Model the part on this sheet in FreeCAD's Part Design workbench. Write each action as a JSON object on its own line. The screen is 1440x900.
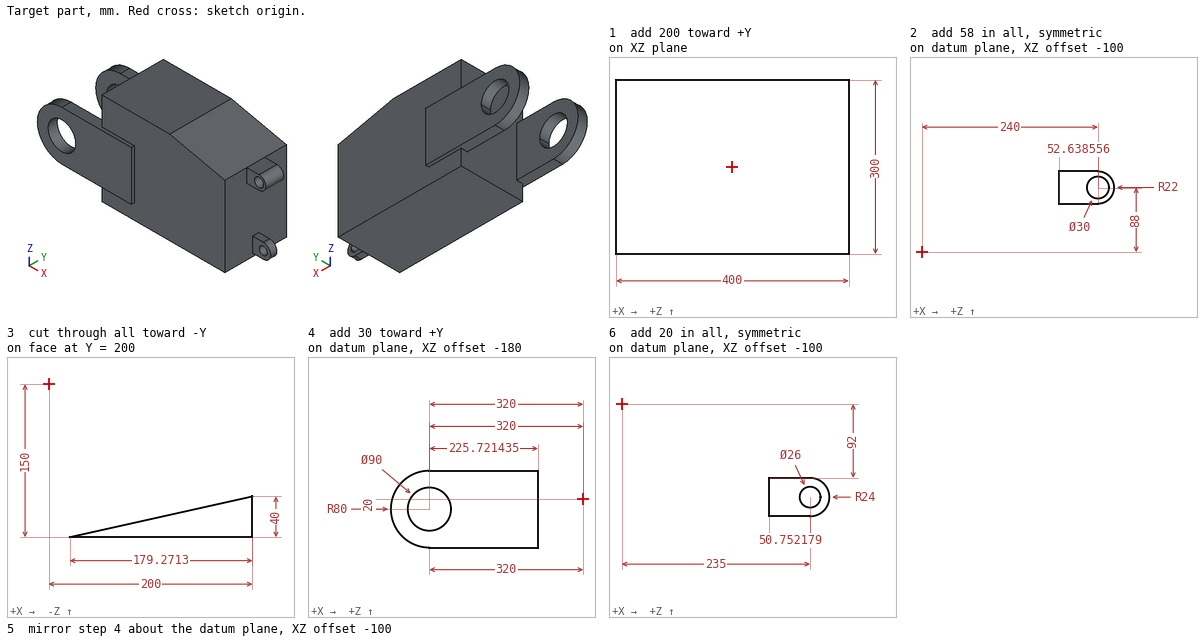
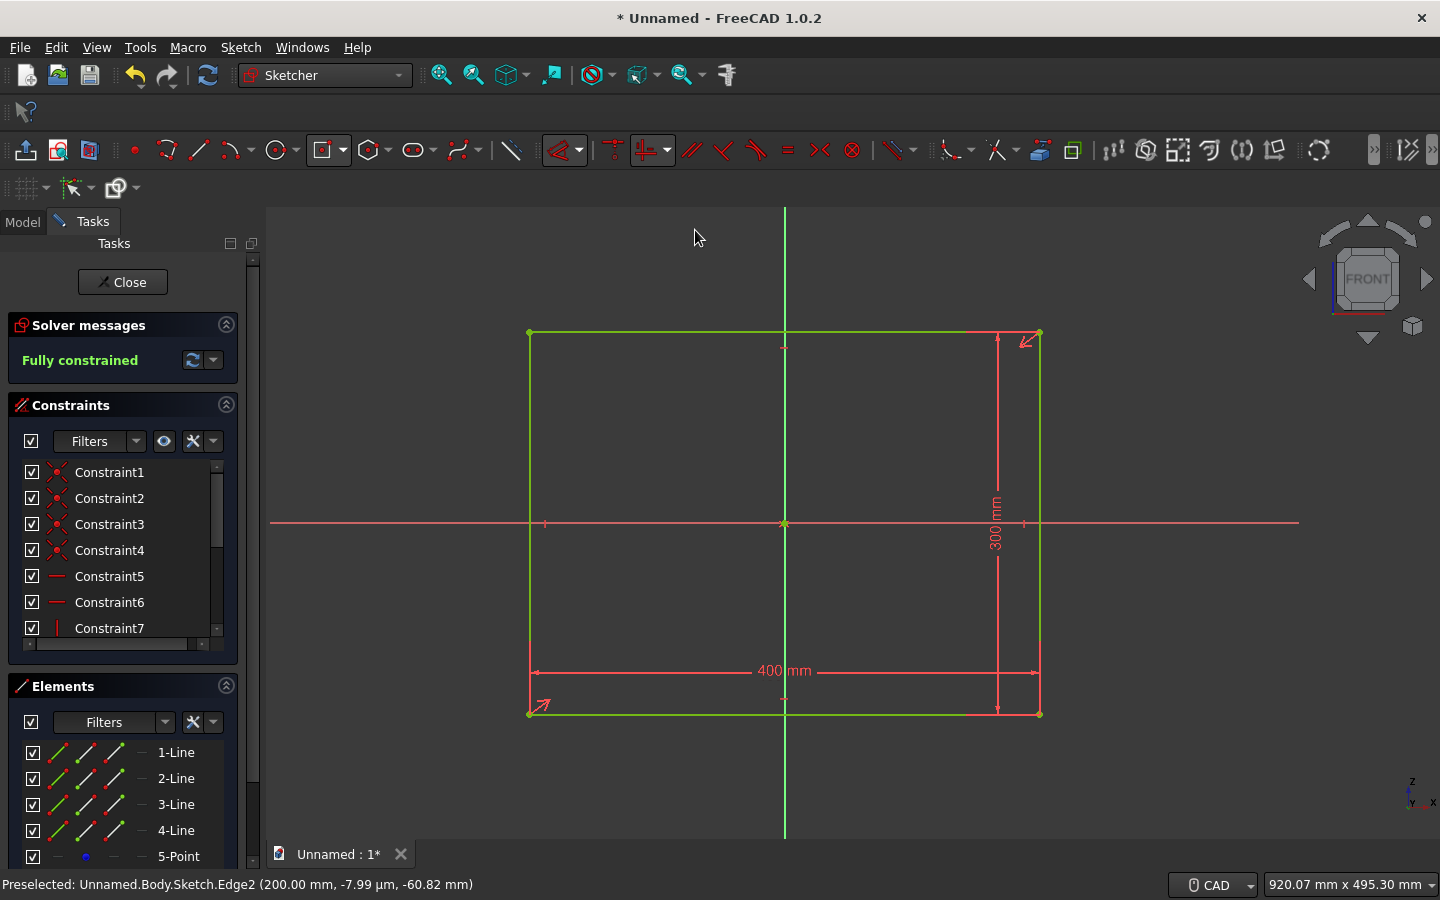
{"action": "left_click", "coordinate": [123, 282]}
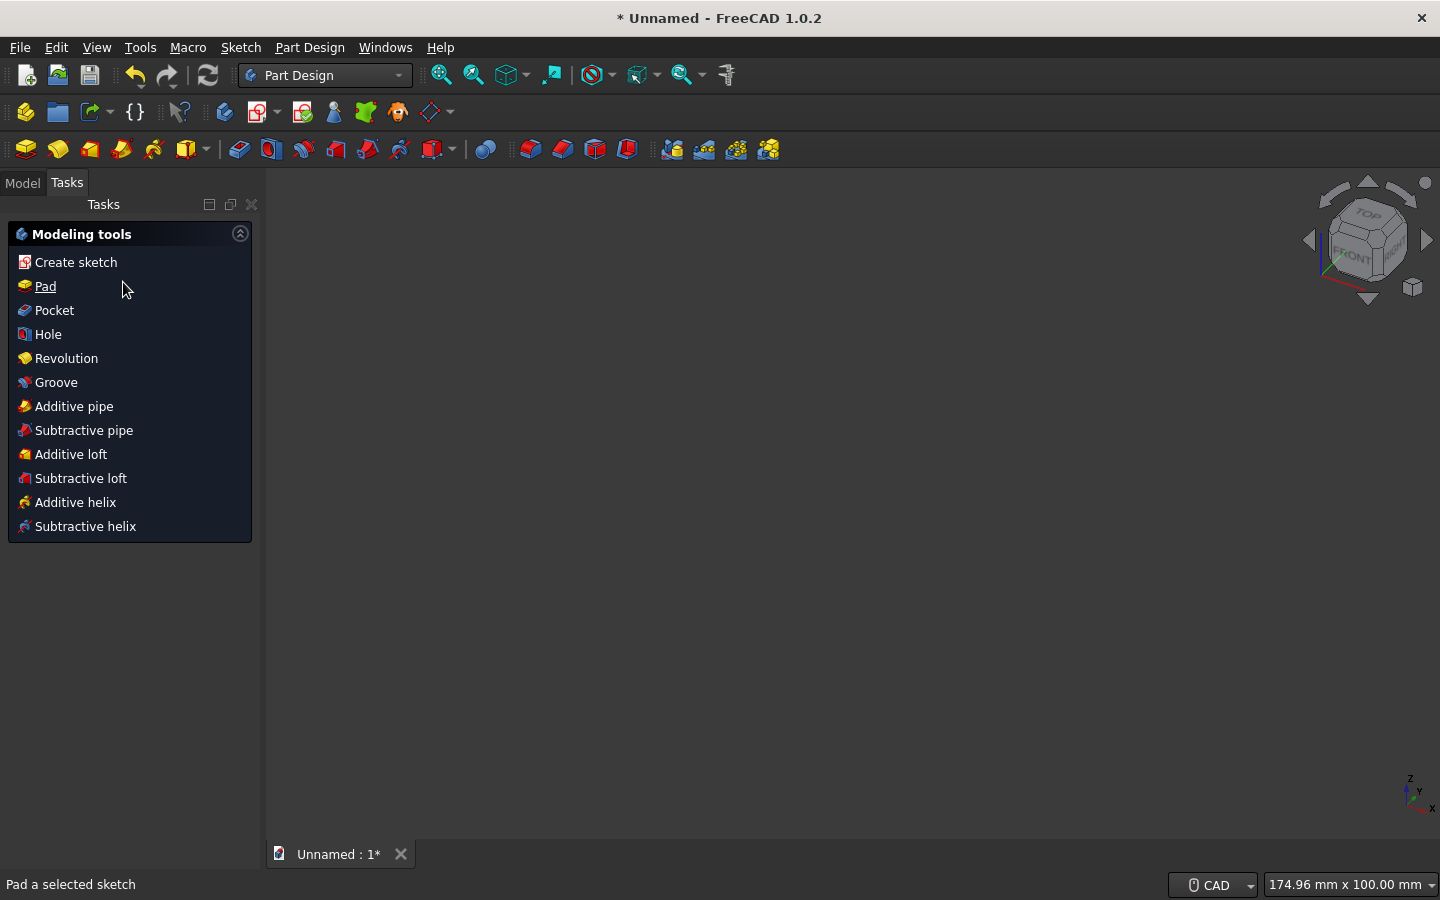
{"action": "left_click", "coordinate": [26, 150]}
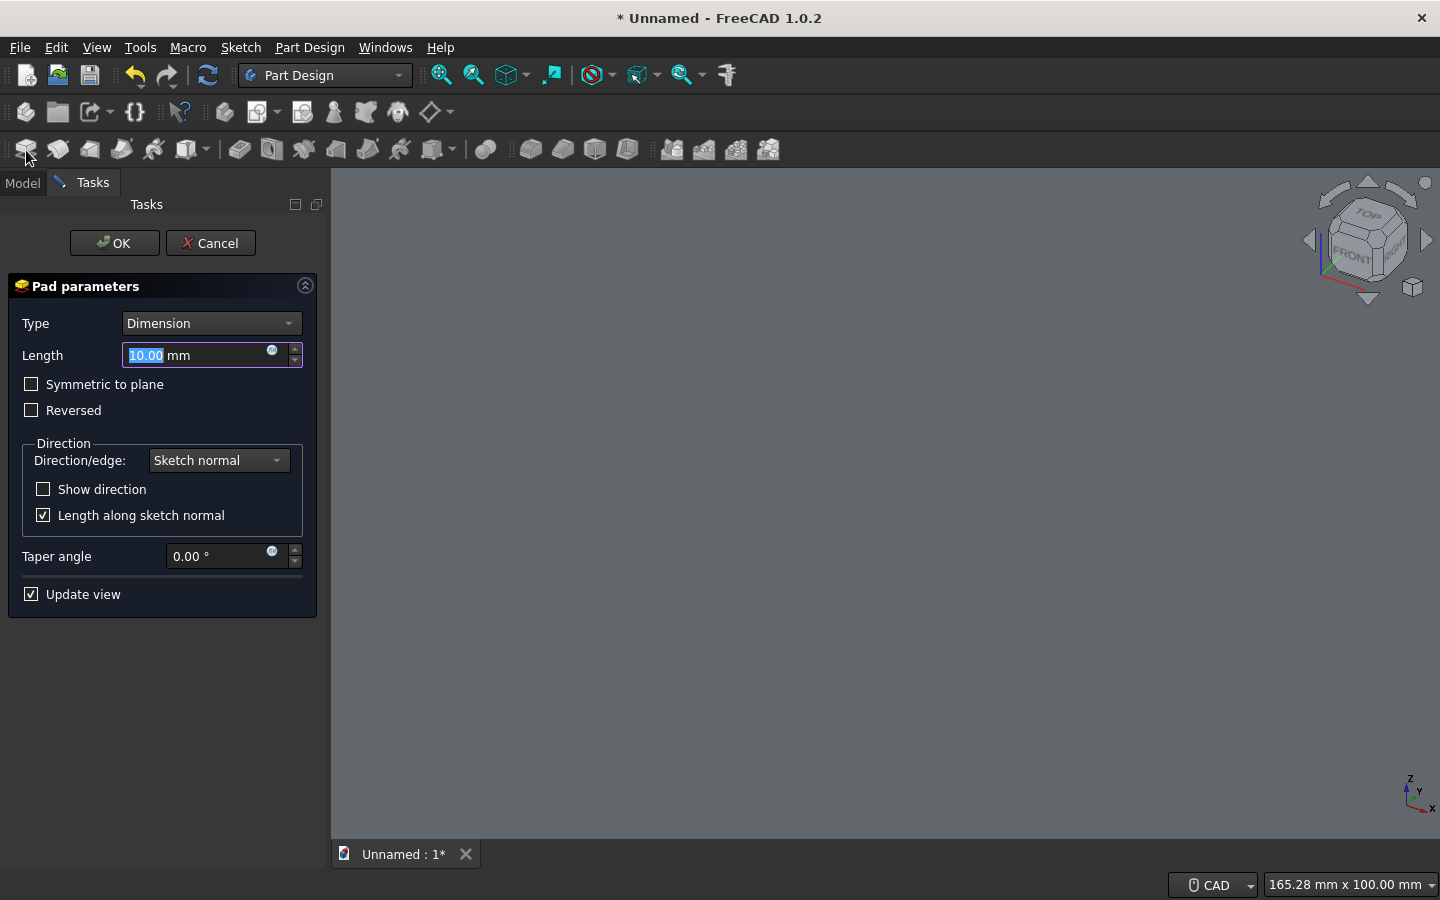
{"action": "type", "text": "200"}
{"action": "key", "text": "Tab"}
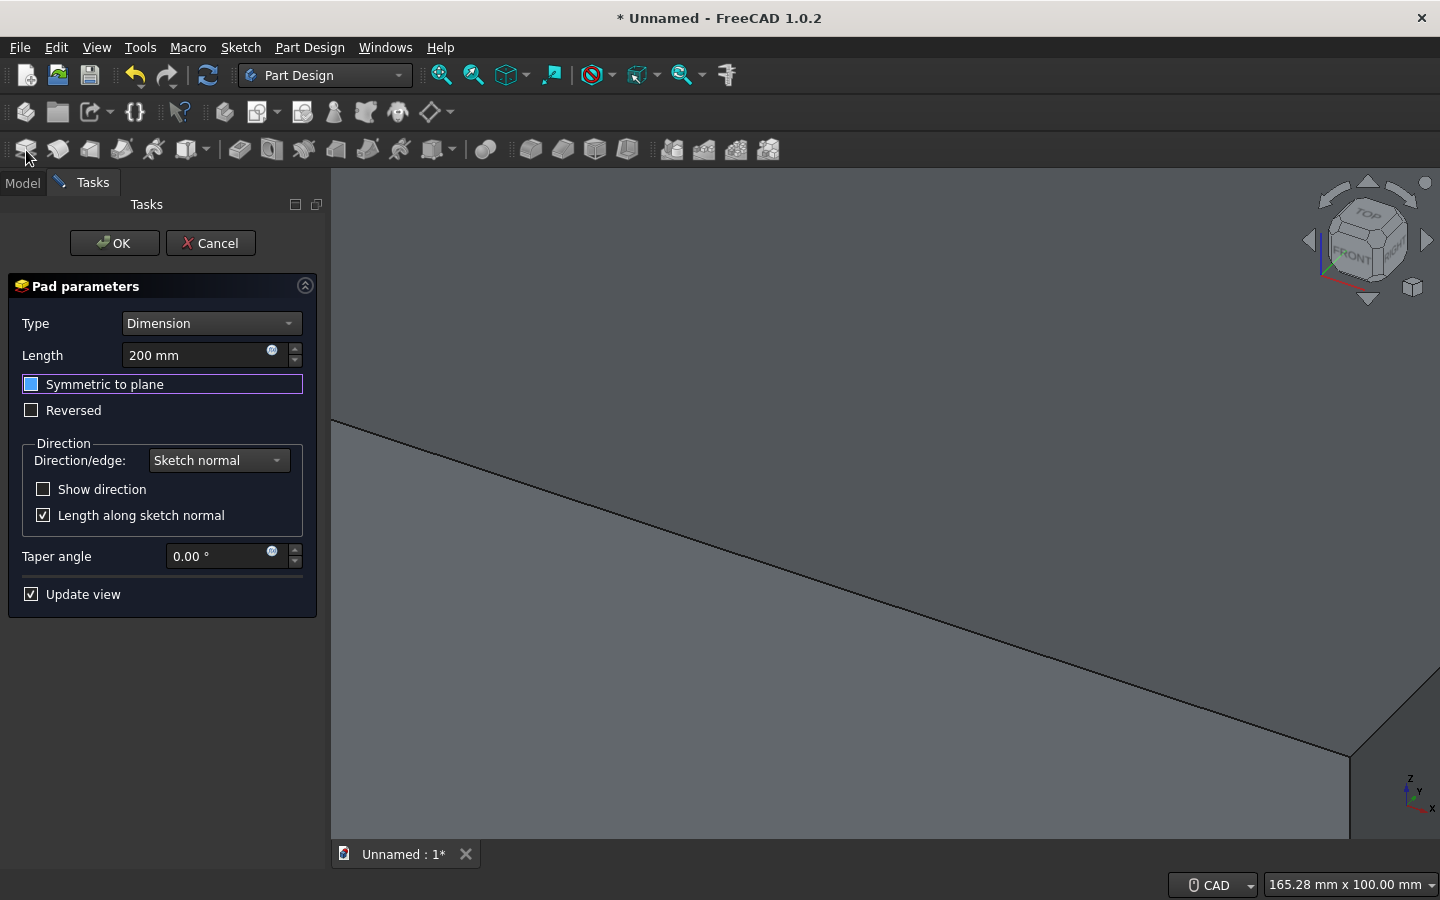
{"action": "left_click", "coordinate": [30, 410]}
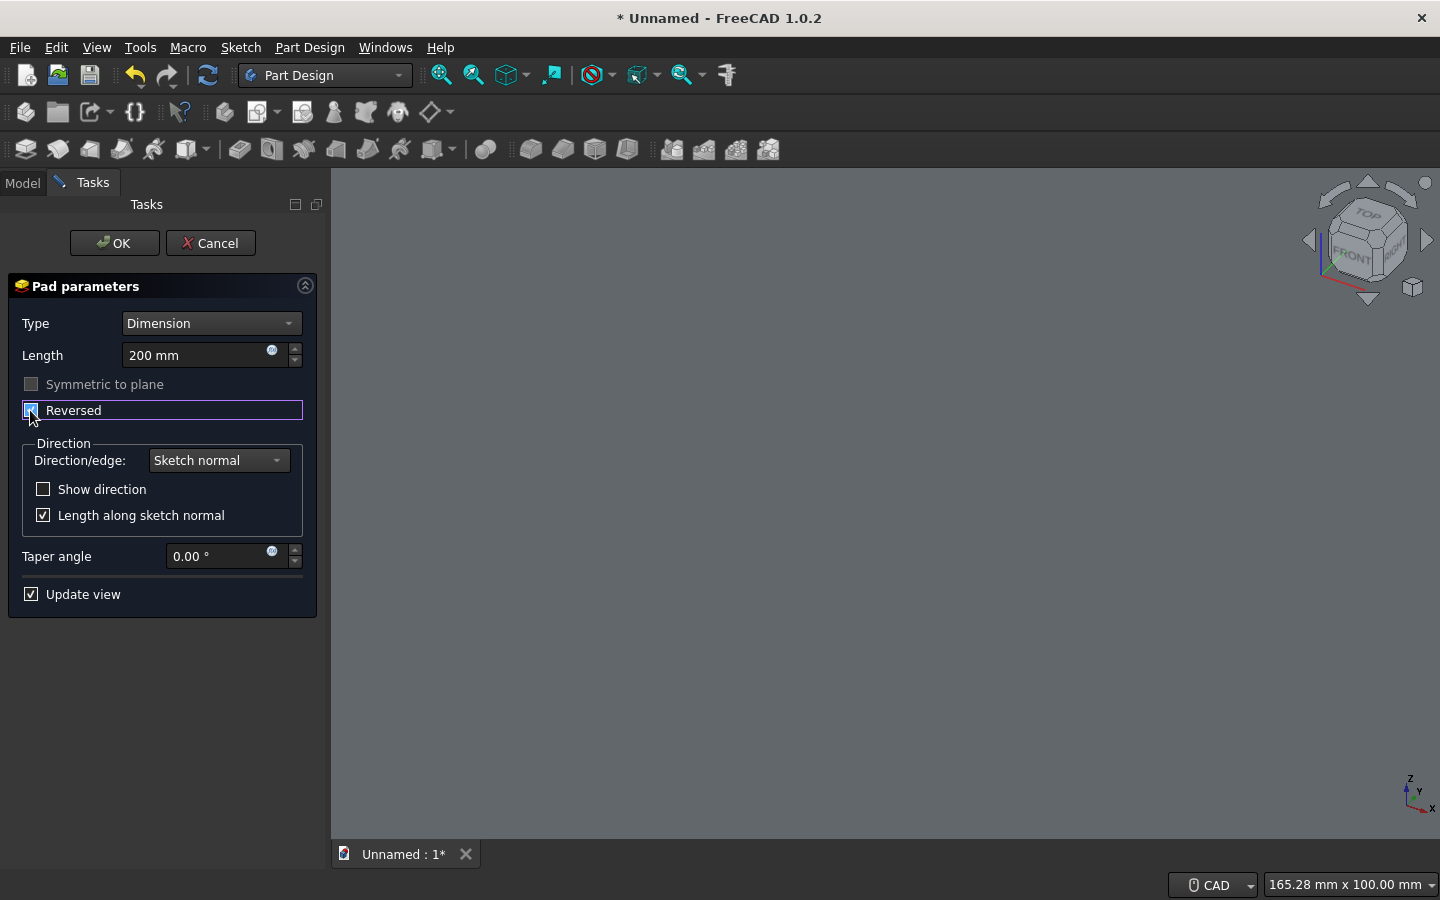
{"action": "left_click", "coordinate": [115, 243]}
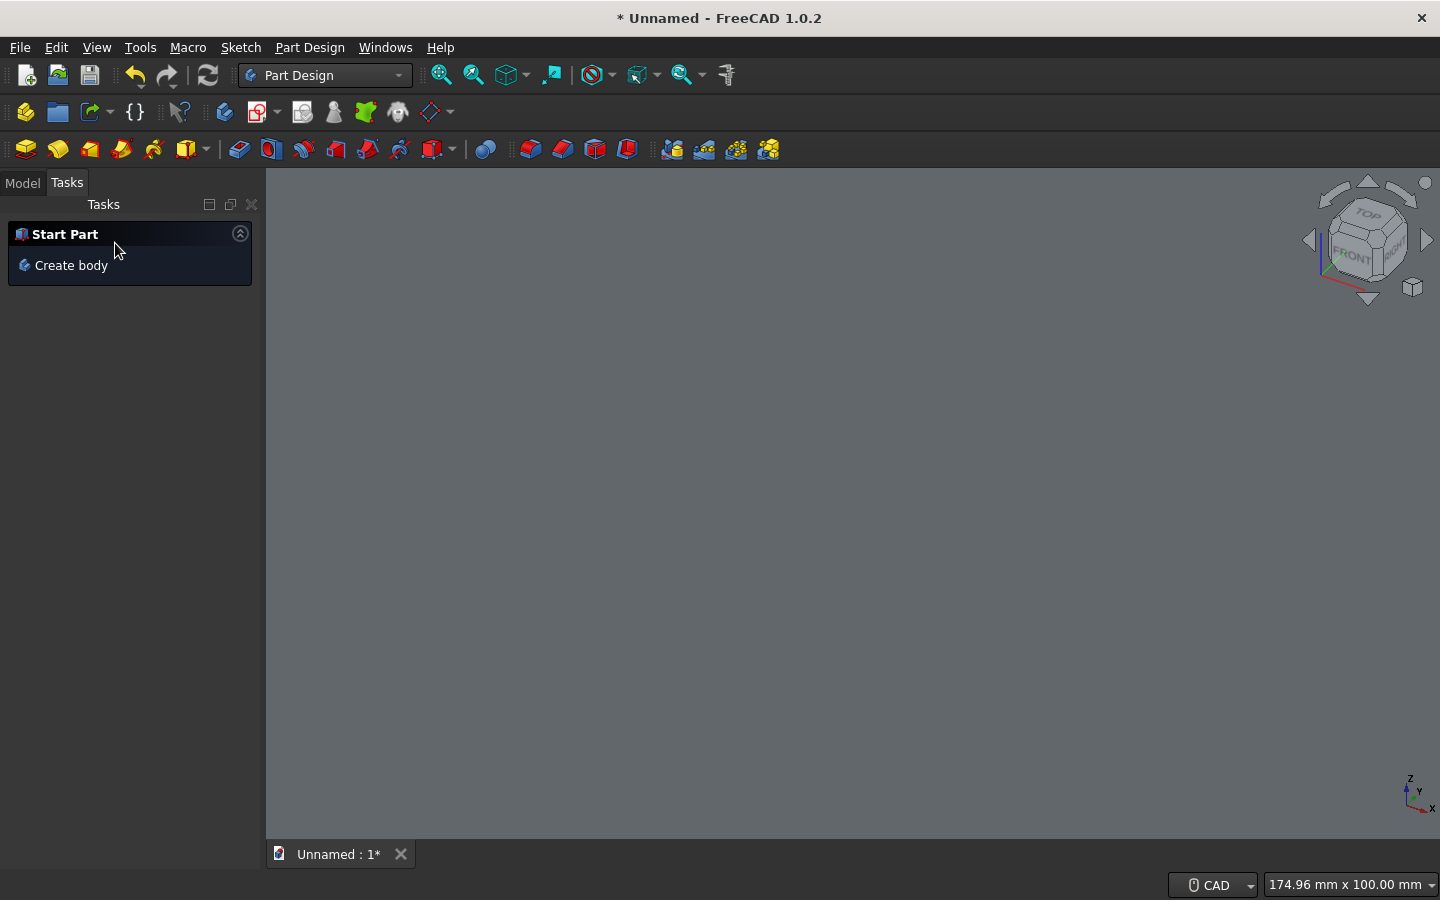
{"action": "left_click", "coordinate": [442, 76]}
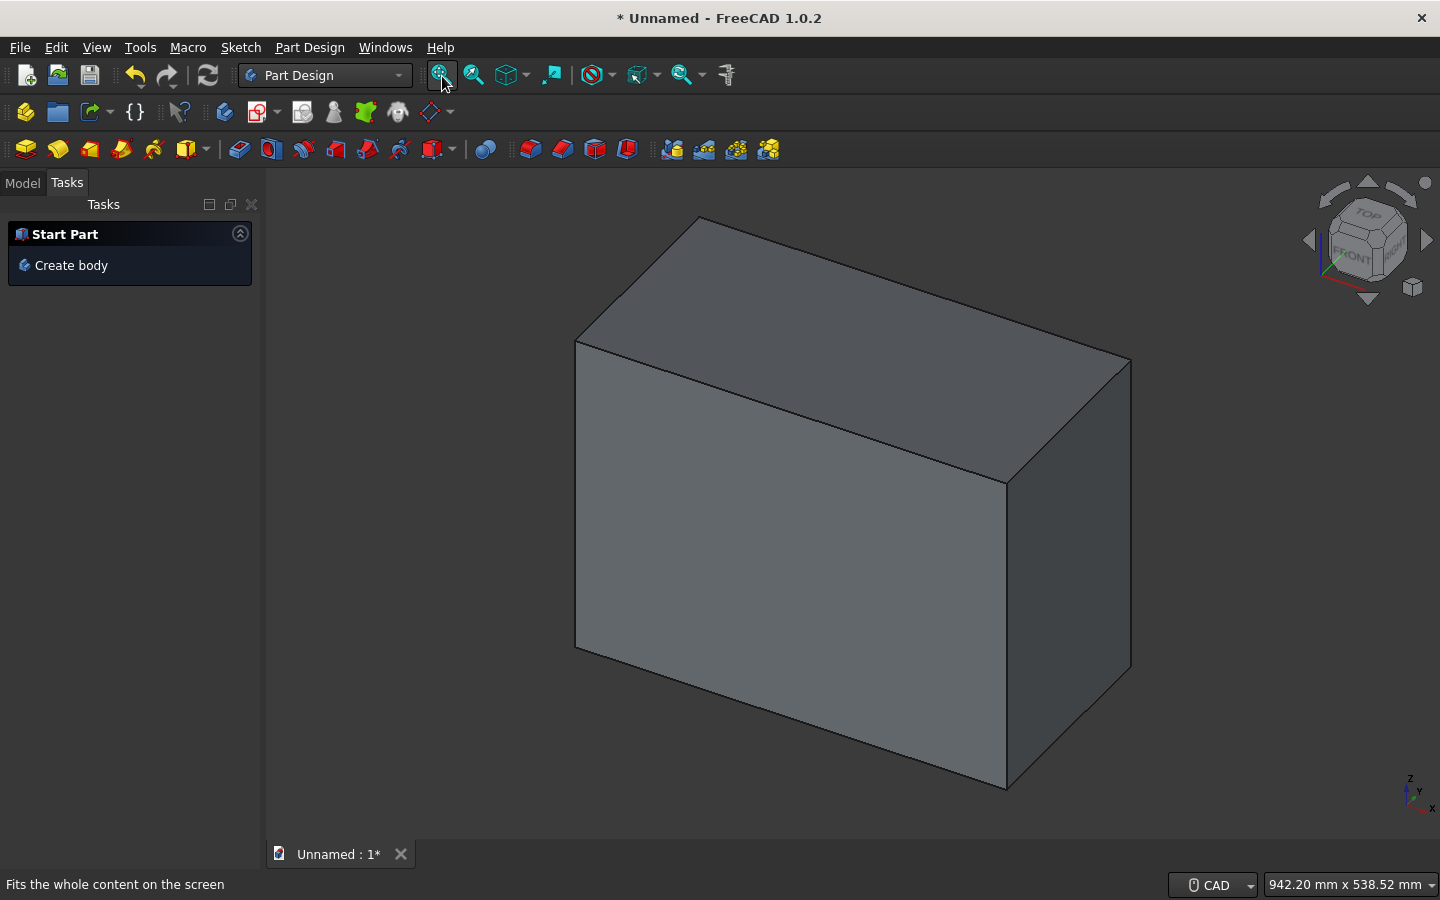
{"action": "left_click", "coordinate": [23, 182]}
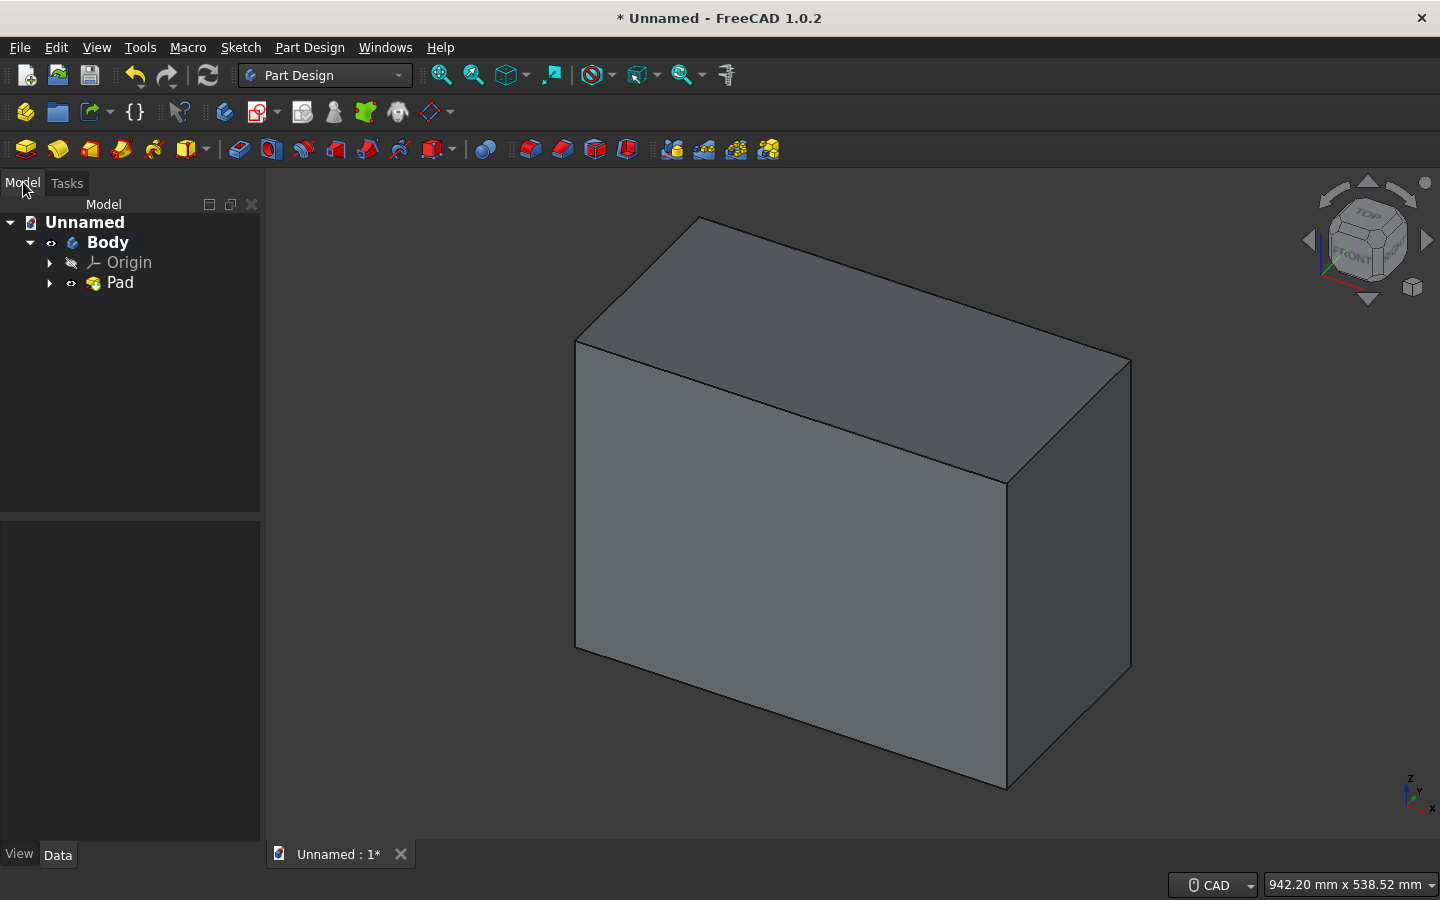
{"action": "left_click", "coordinate": [50, 263]}